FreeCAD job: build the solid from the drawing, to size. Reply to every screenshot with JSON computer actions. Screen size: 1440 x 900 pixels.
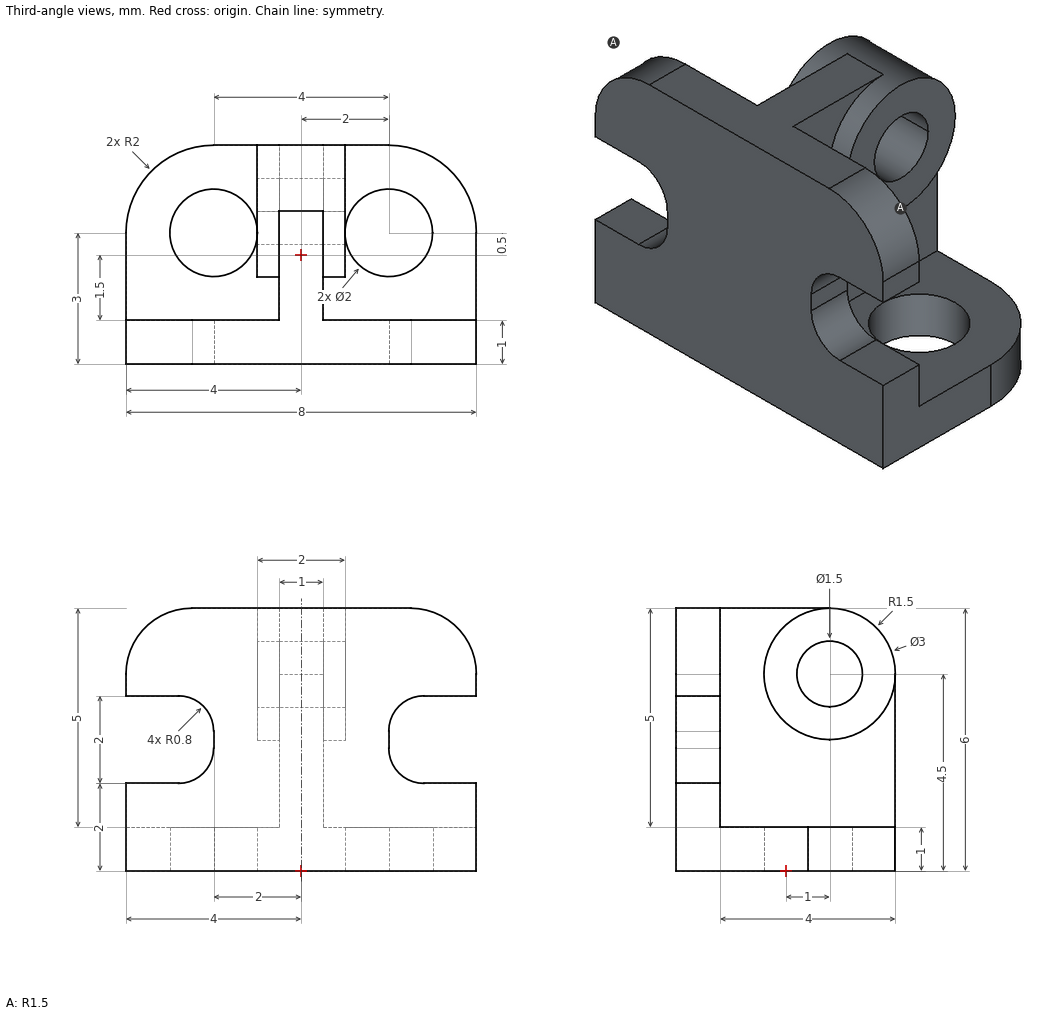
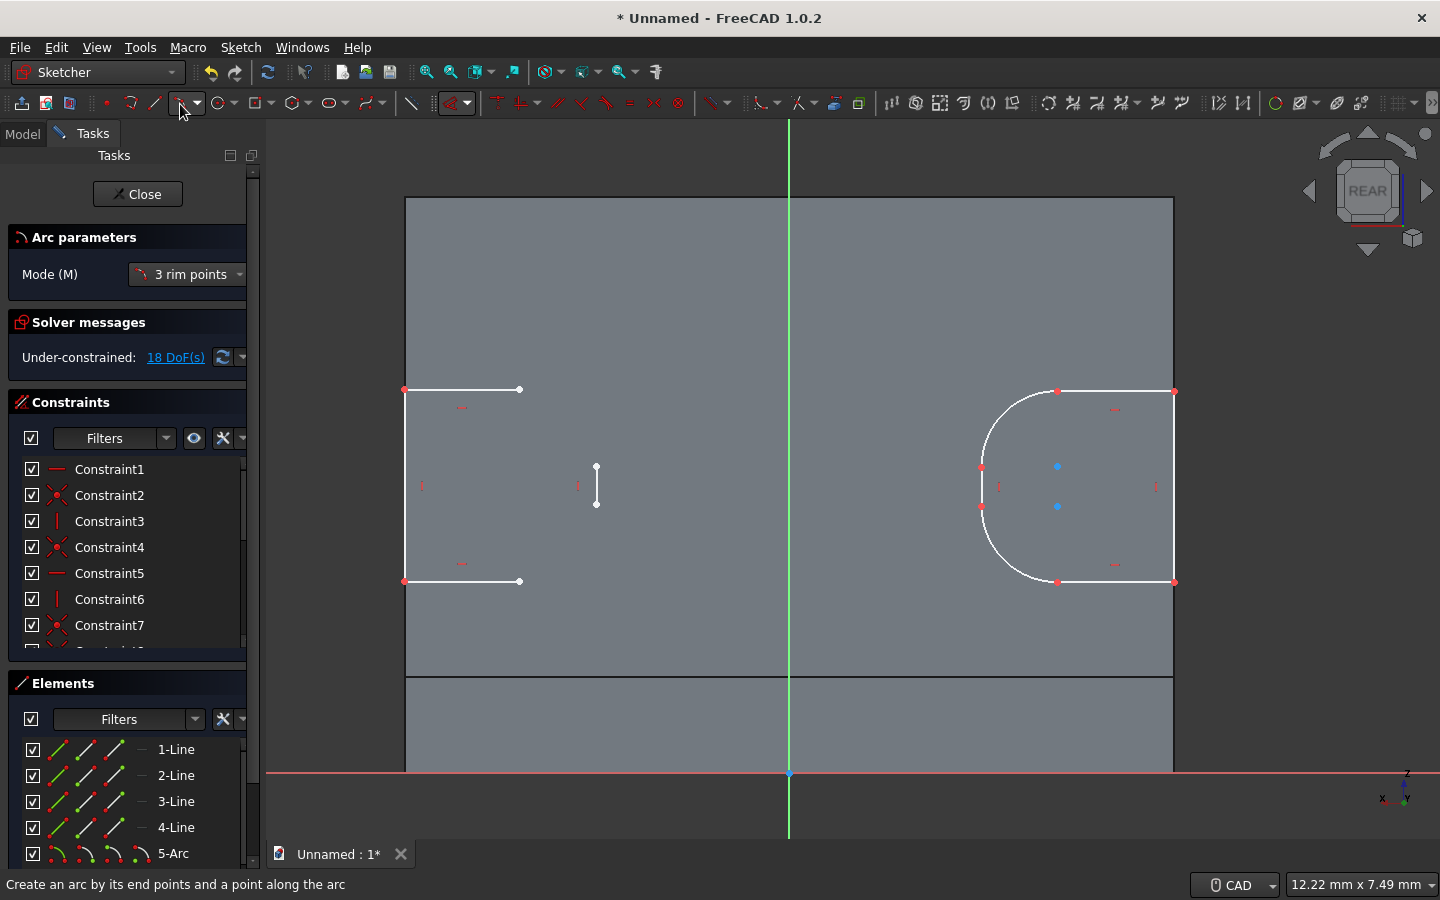
{"action": "left_click", "coordinate": [597, 467]}
{"action": "left_click", "coordinate": [520, 390]}
{"action": "left_click", "coordinate": [575, 412]}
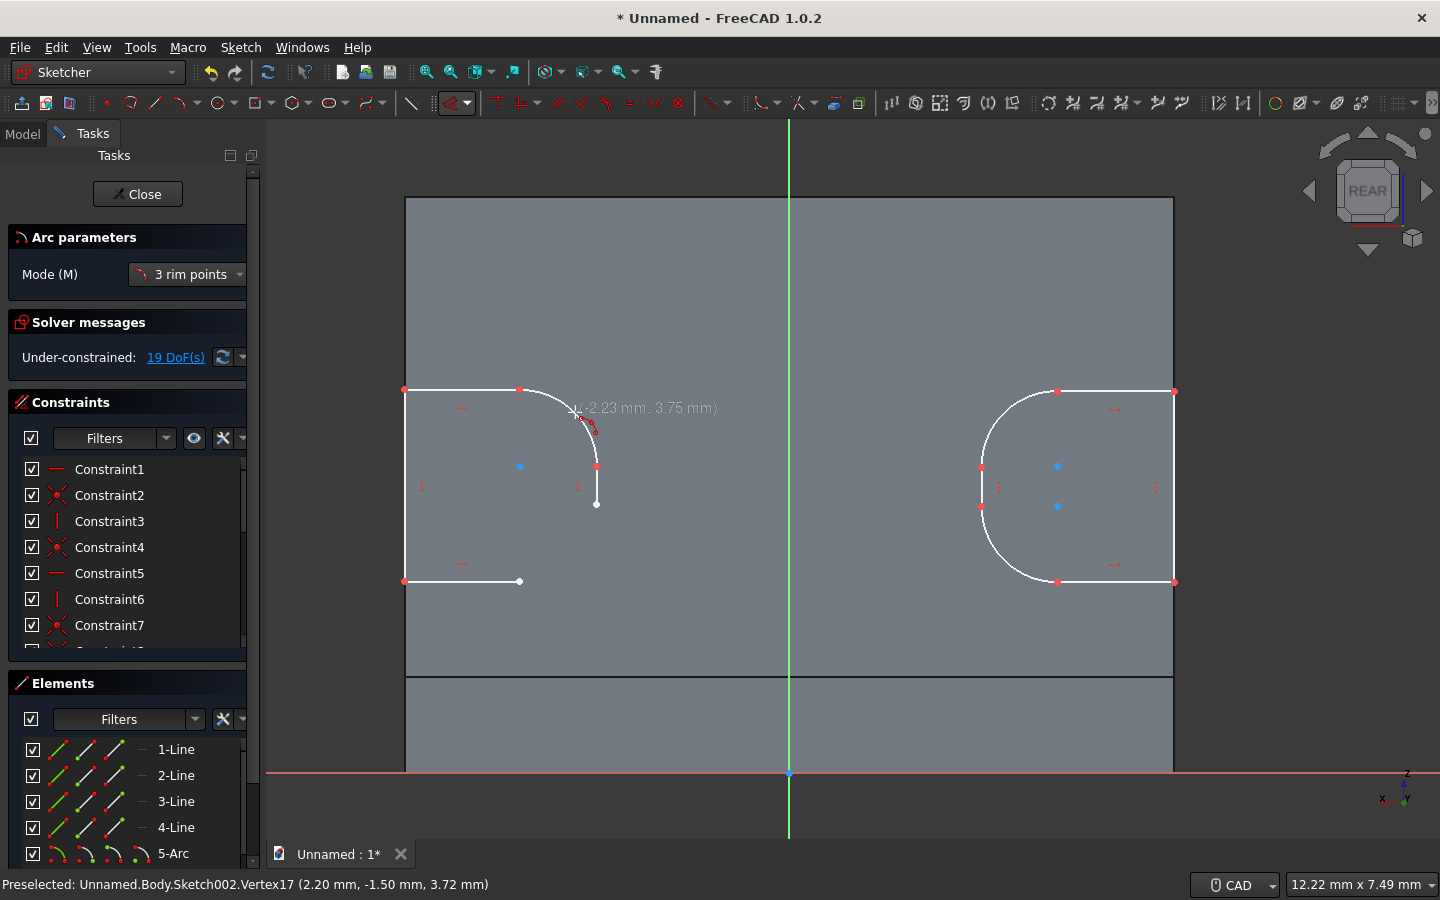
{"action": "left_click", "coordinate": [520, 582]}
{"action": "left_click", "coordinate": [597, 505]}
{"action": "left_click", "coordinate": [575, 559]}
{"action": "key", "text": "Escape"}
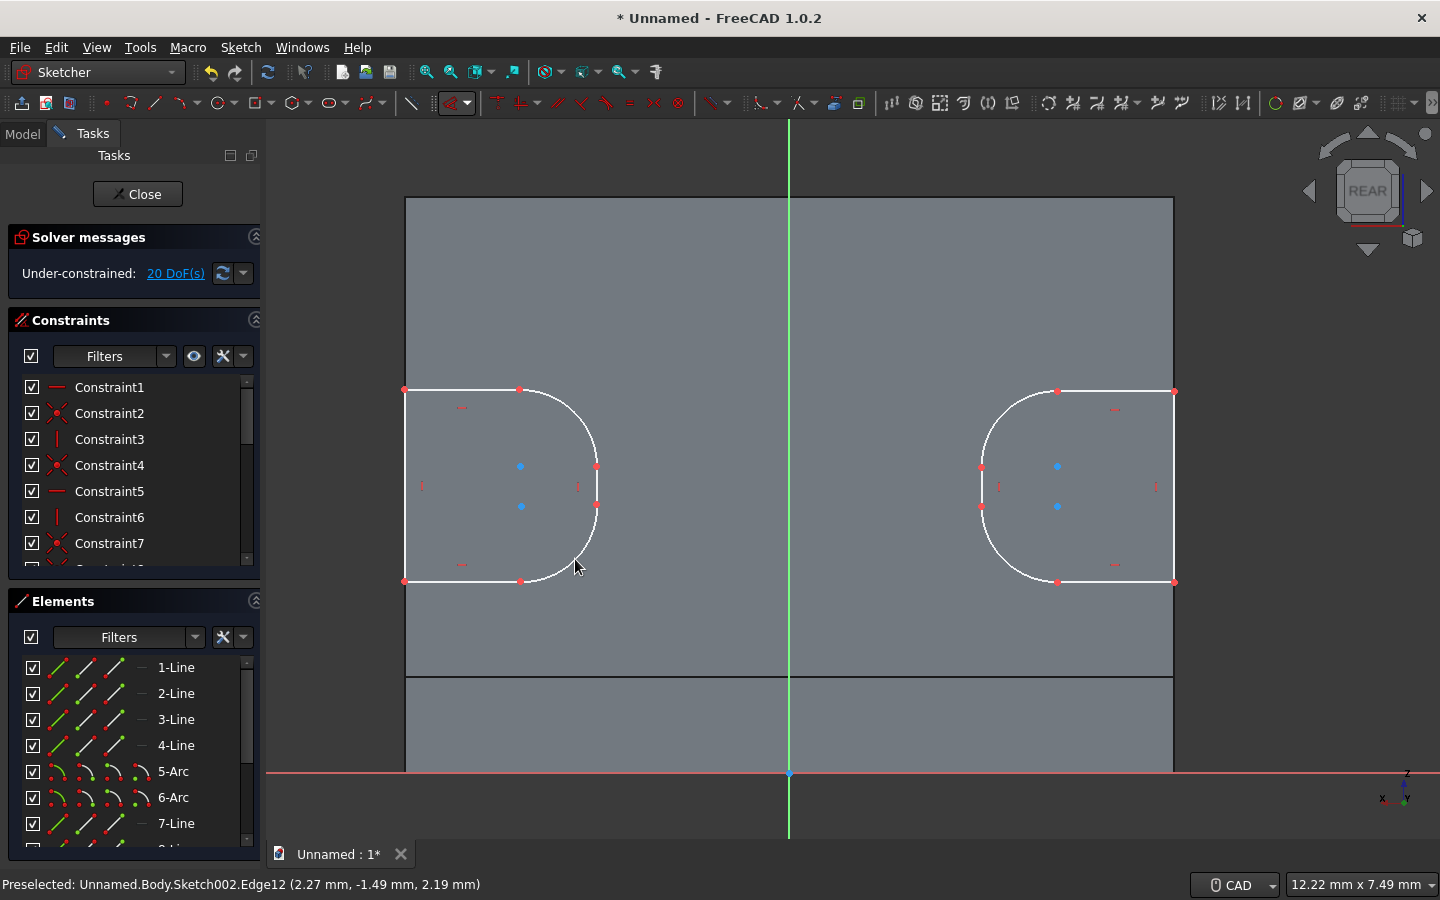
{"action": "left_click", "coordinate": [1093, 582]}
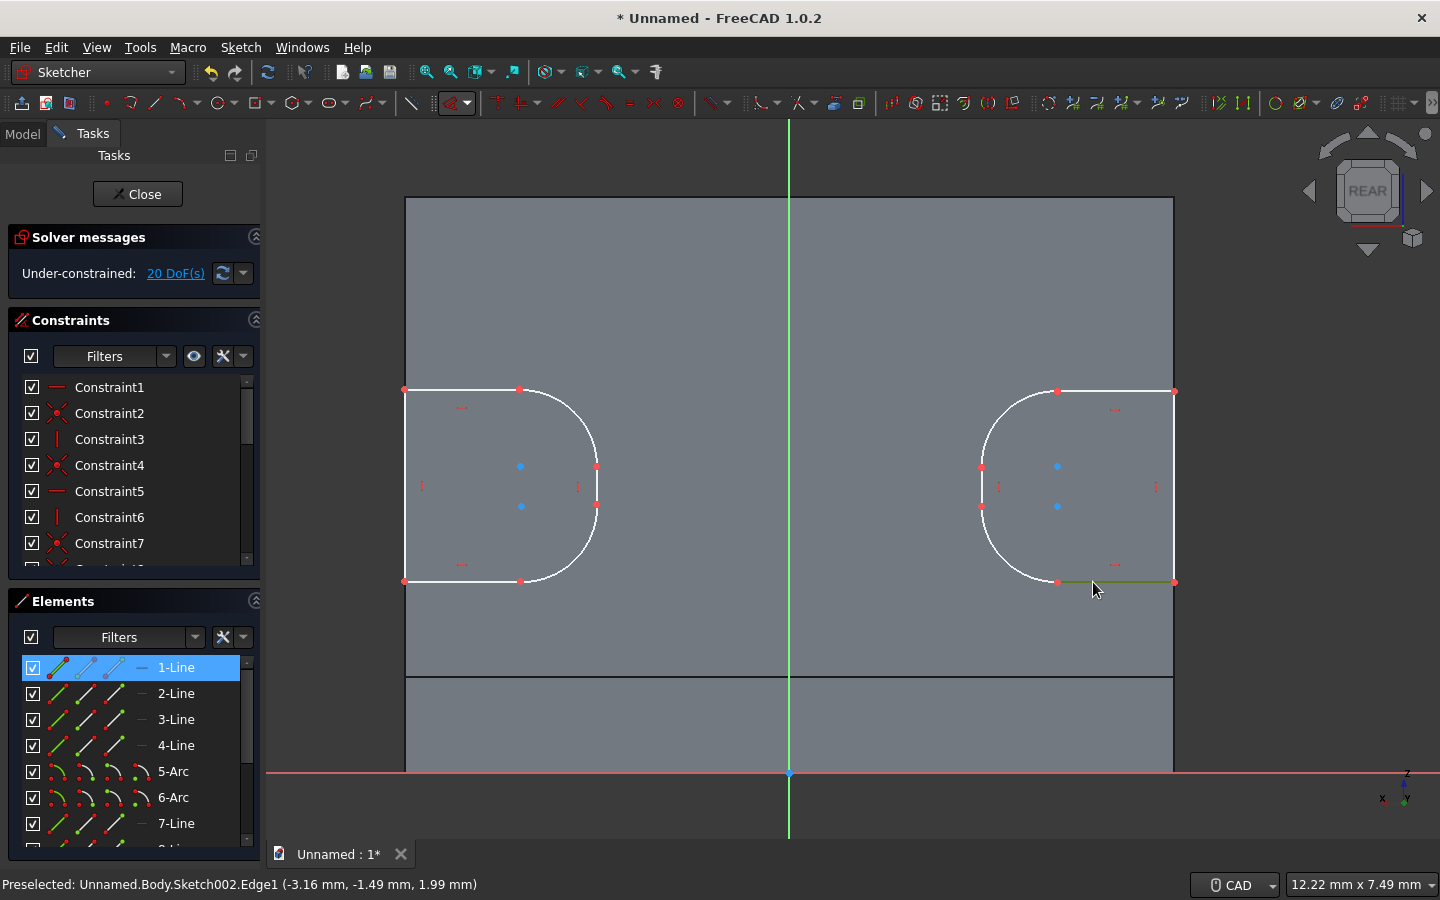
{"action": "left_click", "coordinate": [990, 541]}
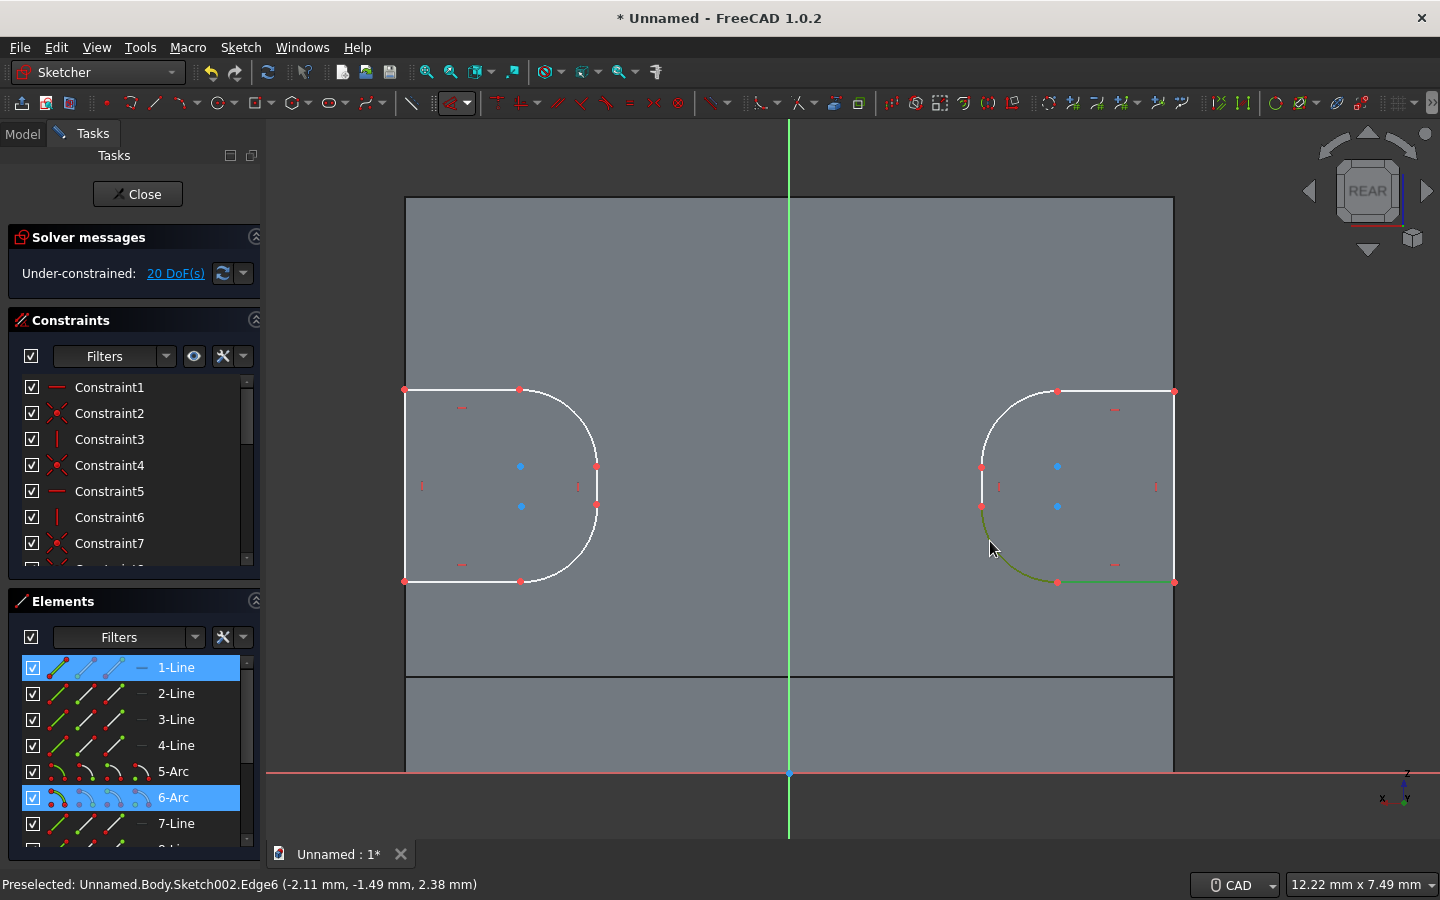
{"action": "left_click", "coordinate": [606, 104]}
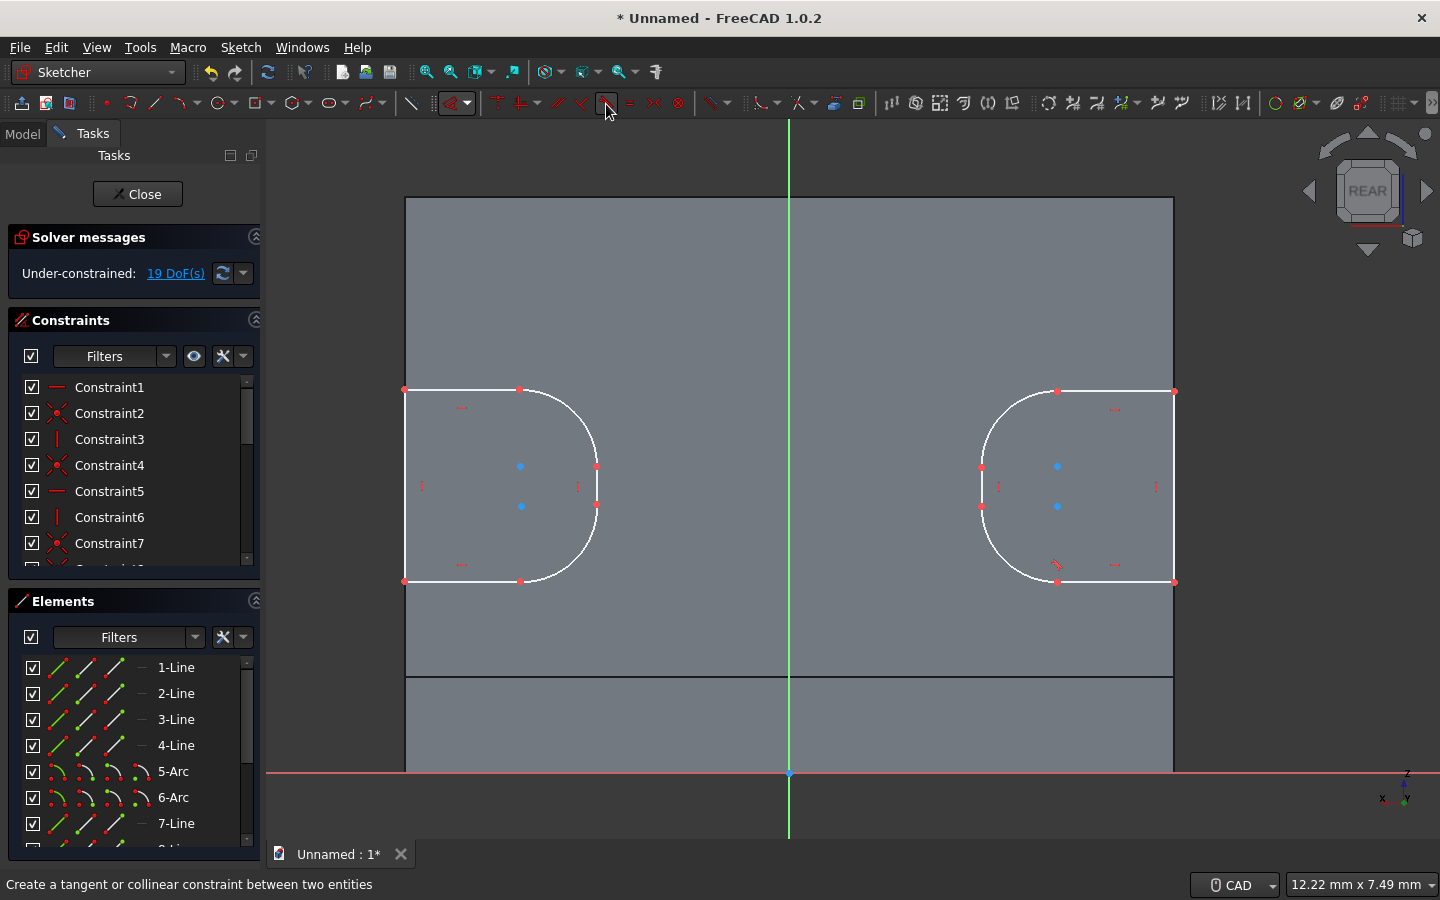
{"action": "left_click", "coordinate": [1139, 391]}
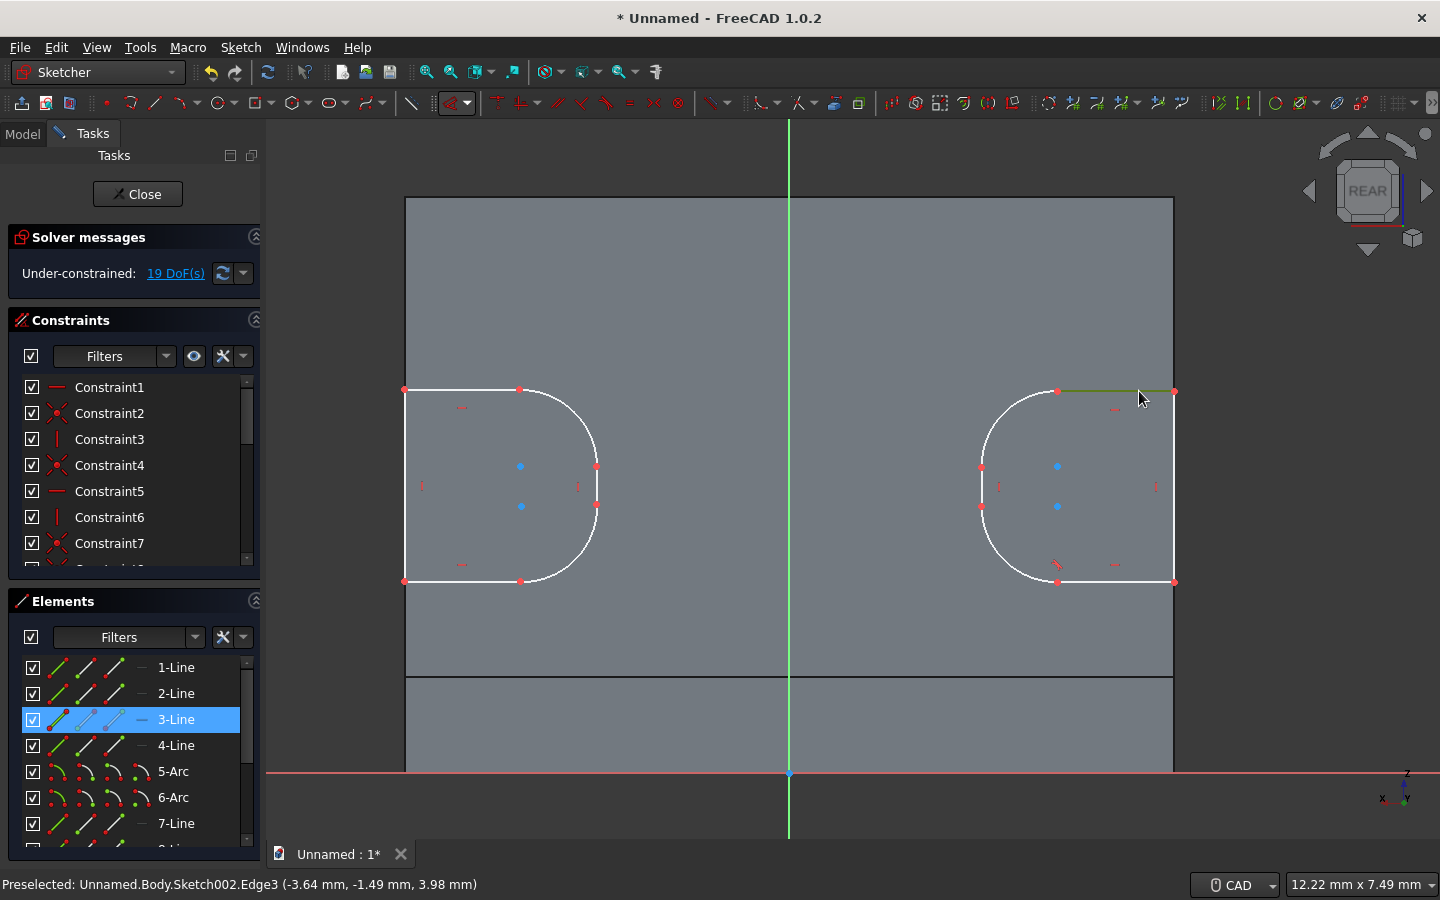
{"action": "left_click", "coordinate": [1023, 399]}